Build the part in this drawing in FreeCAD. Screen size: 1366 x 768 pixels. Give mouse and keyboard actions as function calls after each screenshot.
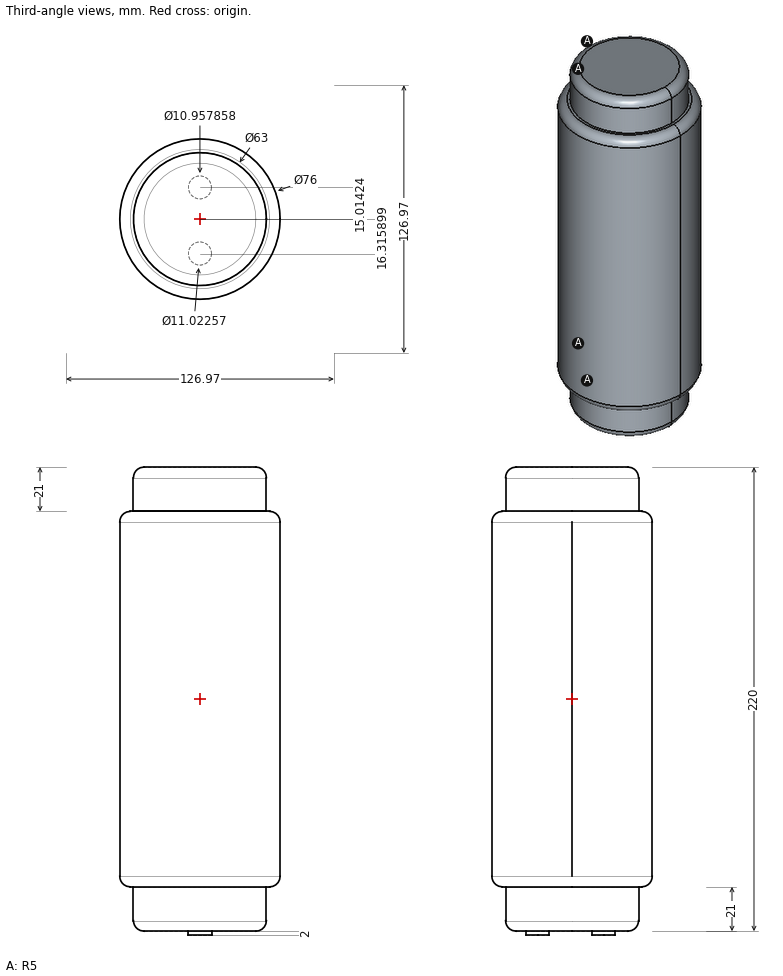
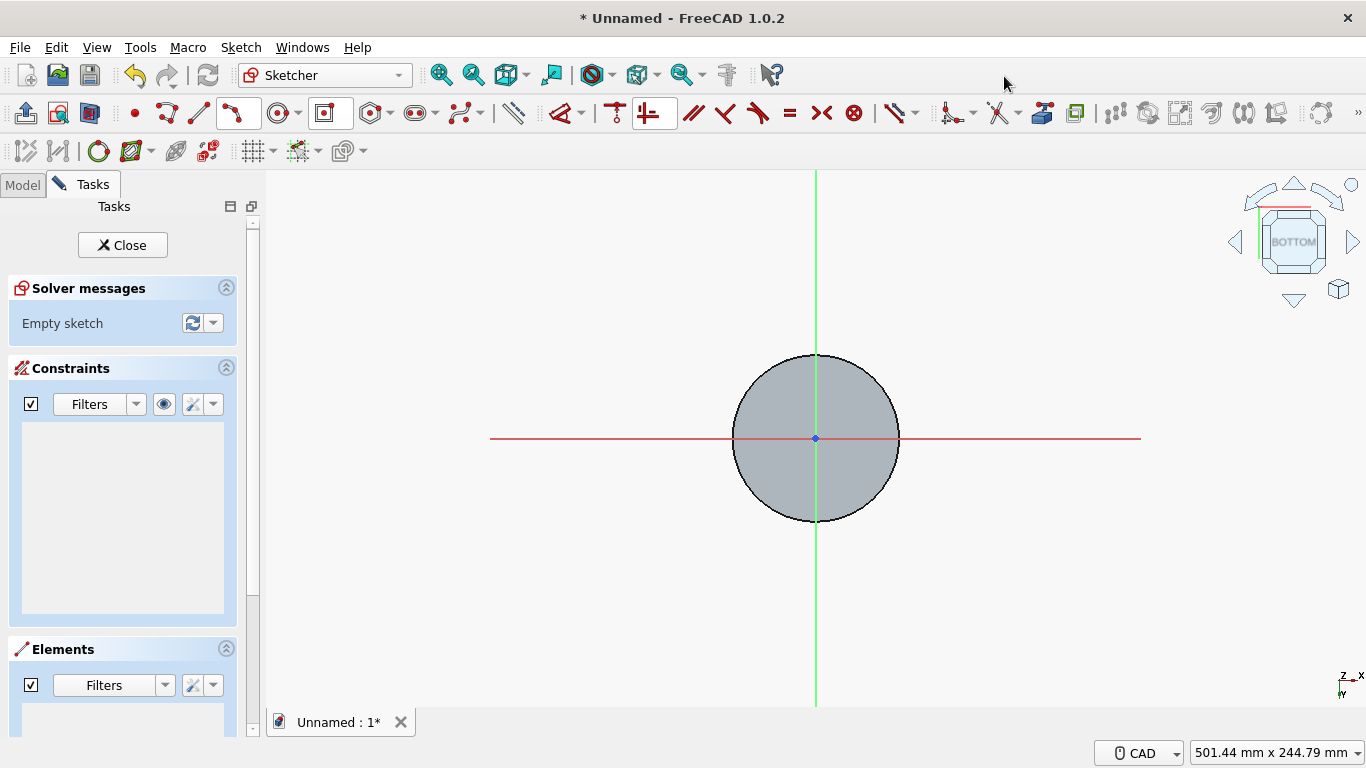
click(324, 114)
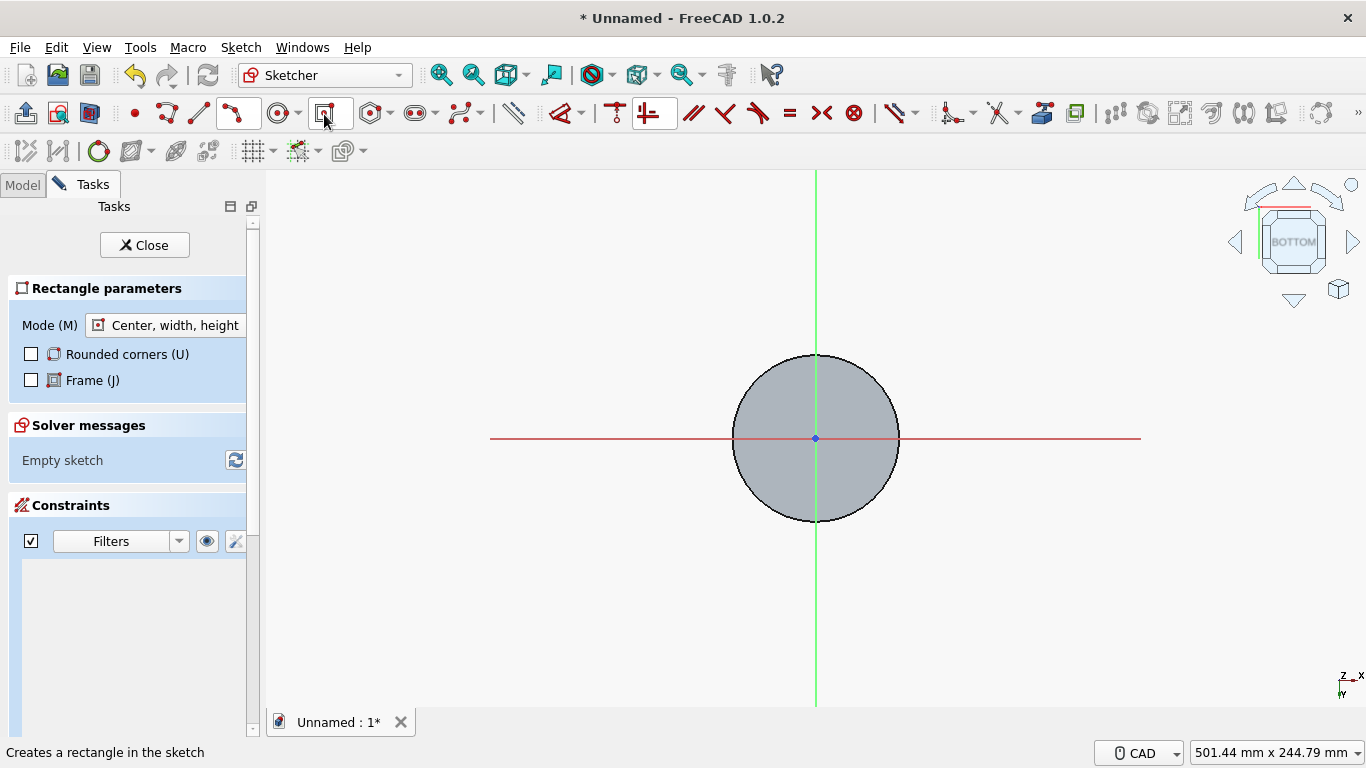
click(816, 438)
move(955, 299)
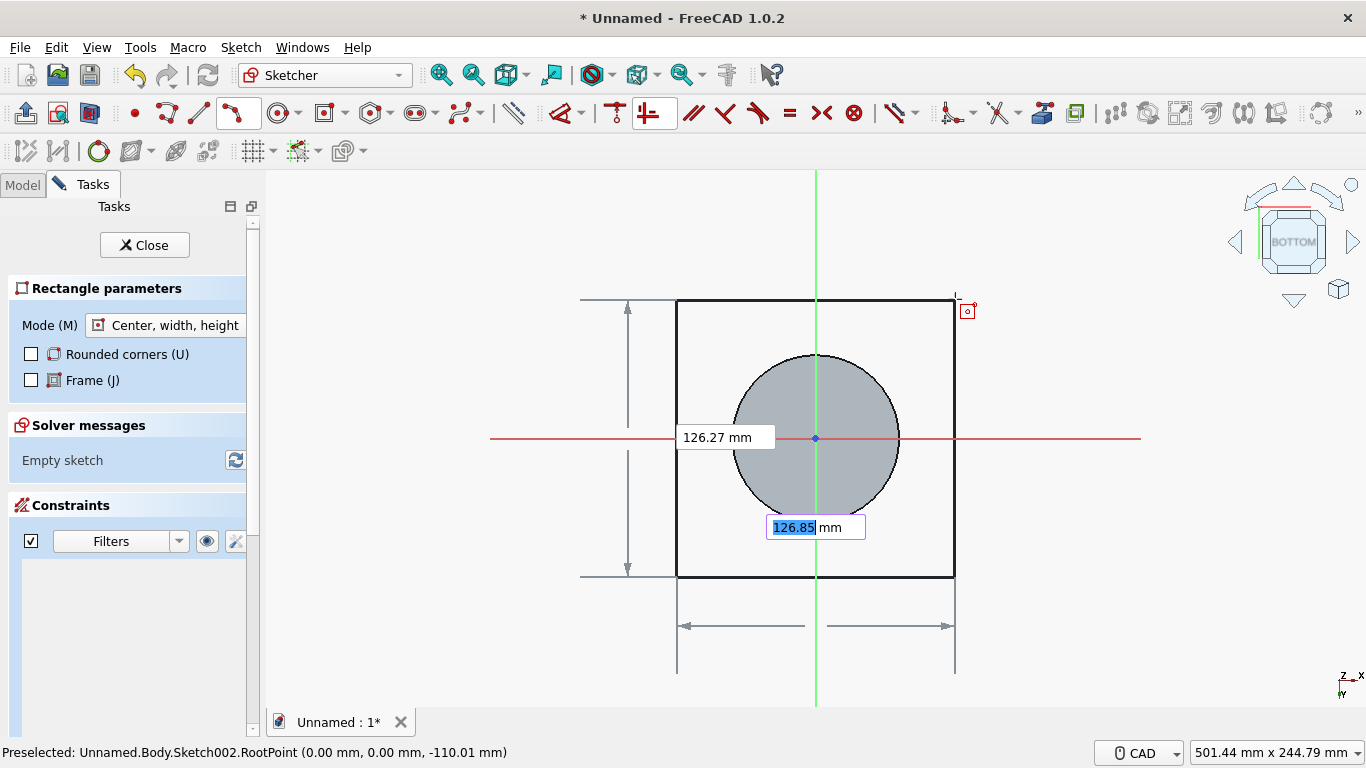
text(126.97)
key(Tab)
text(126.97)
key(Return)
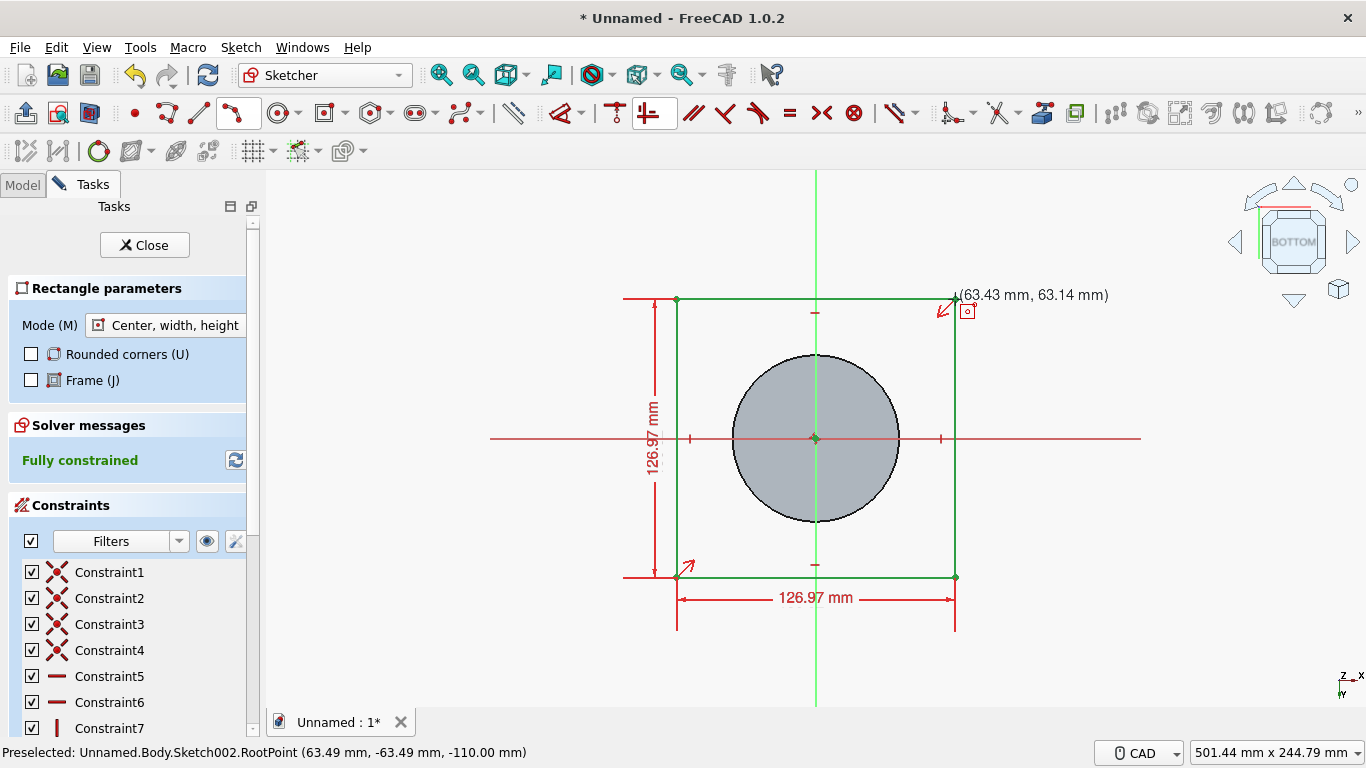
click(278, 114)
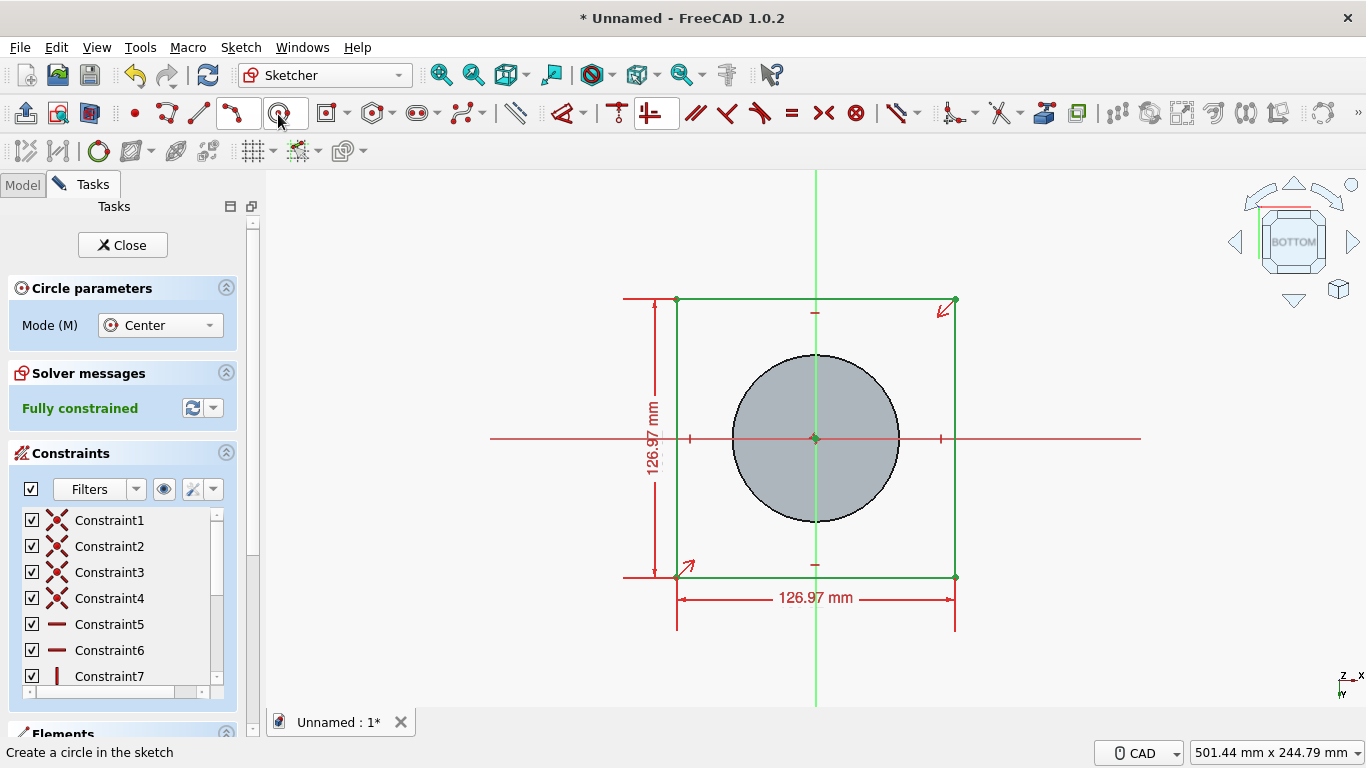
click(816, 438)
move(865, 390)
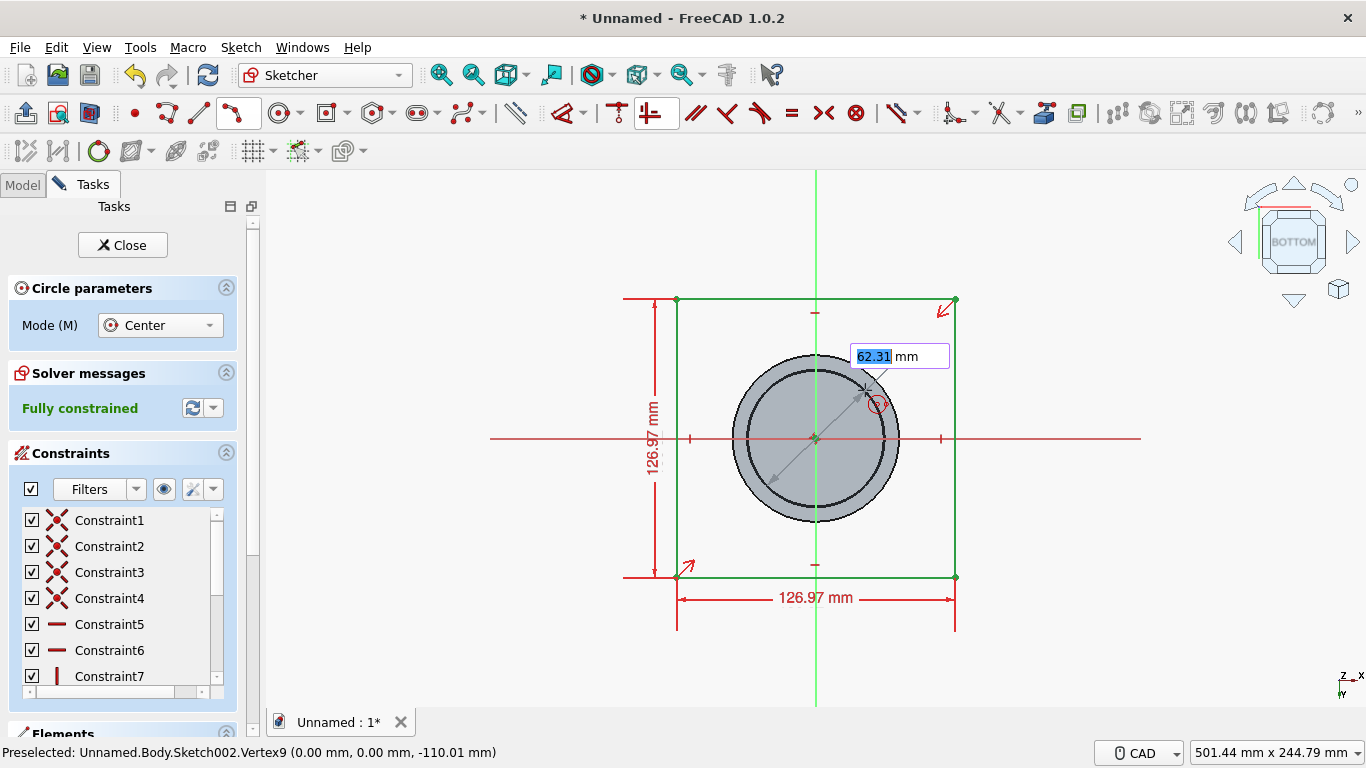
text(63)
key(Return)
key(Escape)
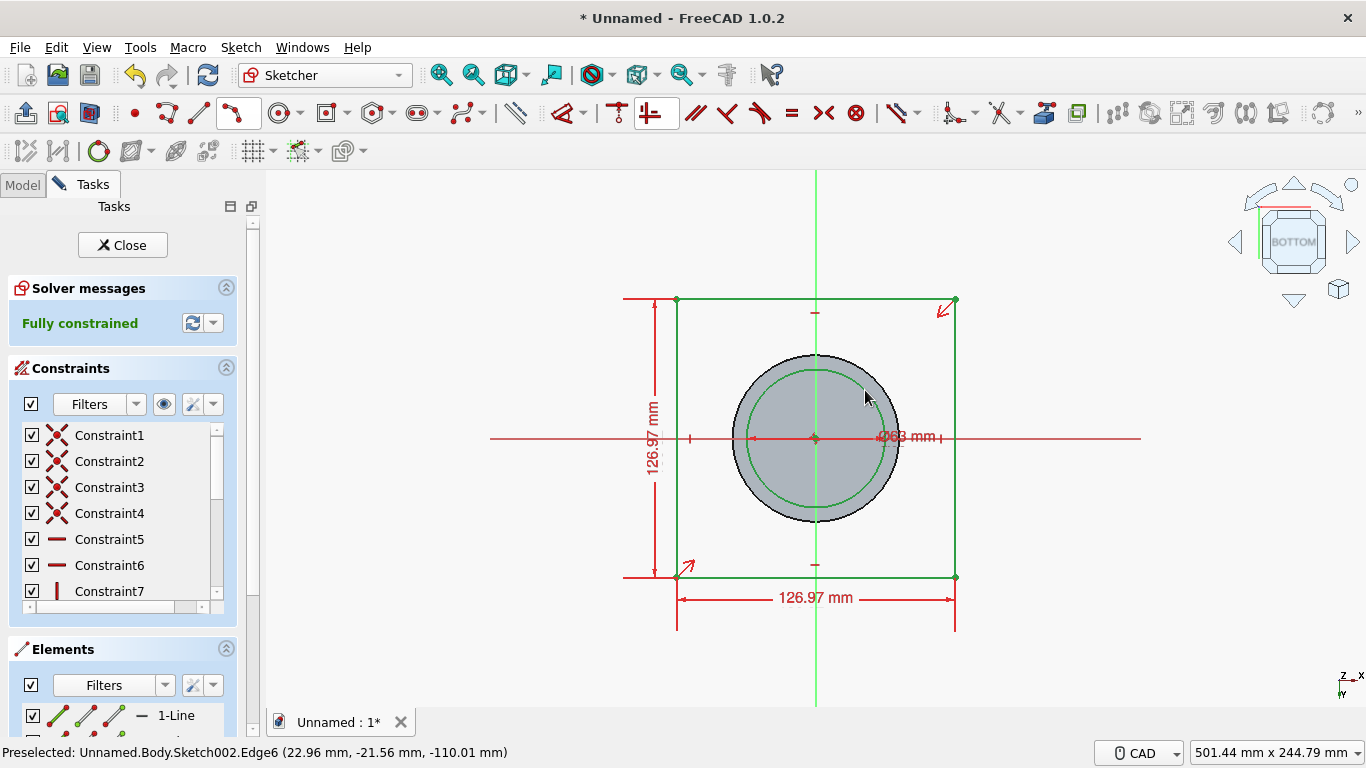
click(123, 245)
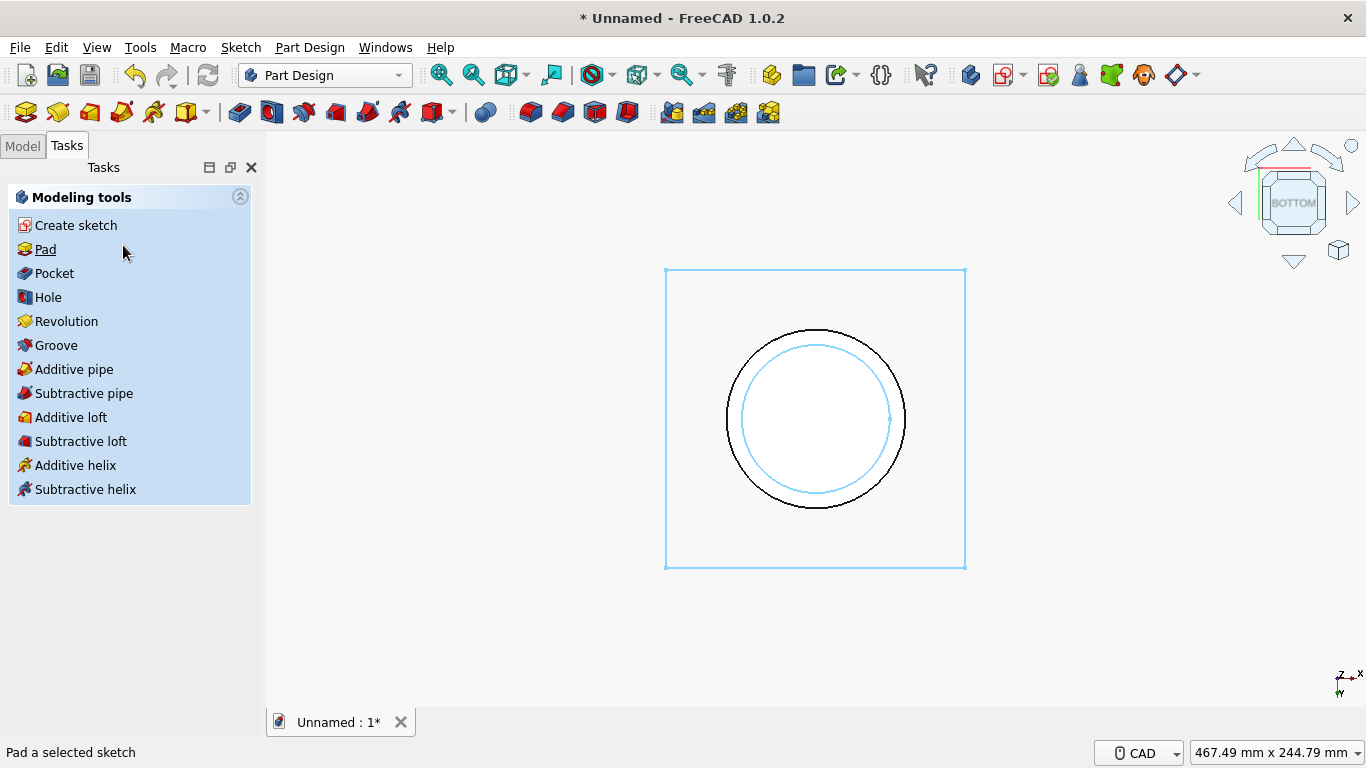
click(240, 112)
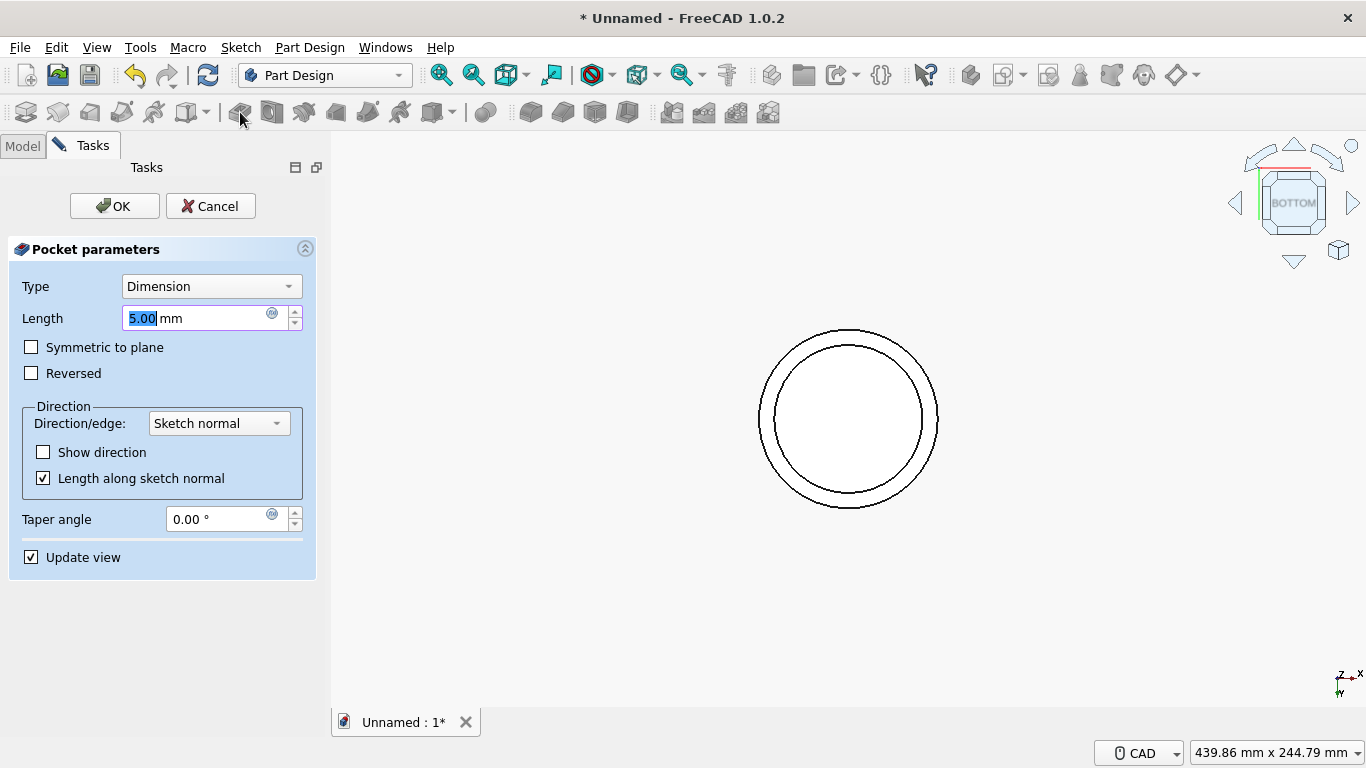
text(21)
key(Tab)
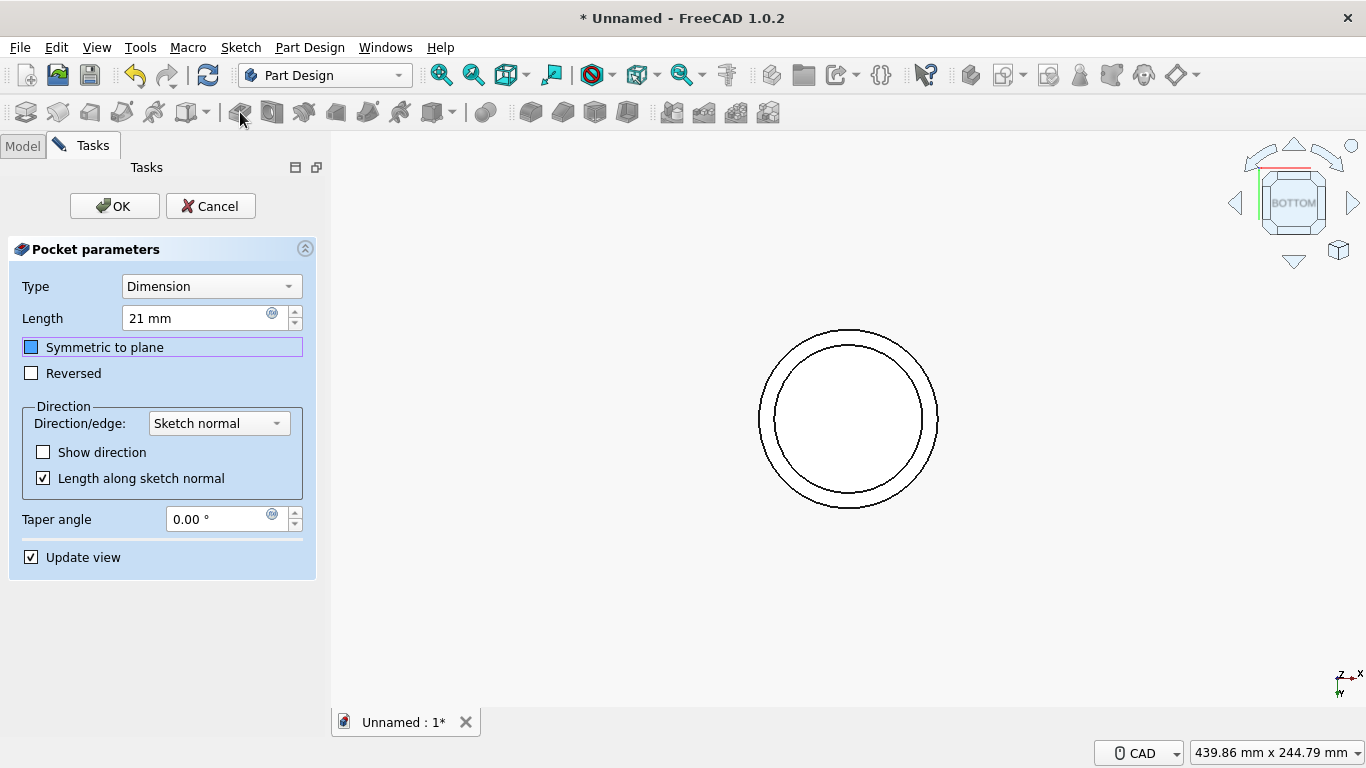
click(115, 206)